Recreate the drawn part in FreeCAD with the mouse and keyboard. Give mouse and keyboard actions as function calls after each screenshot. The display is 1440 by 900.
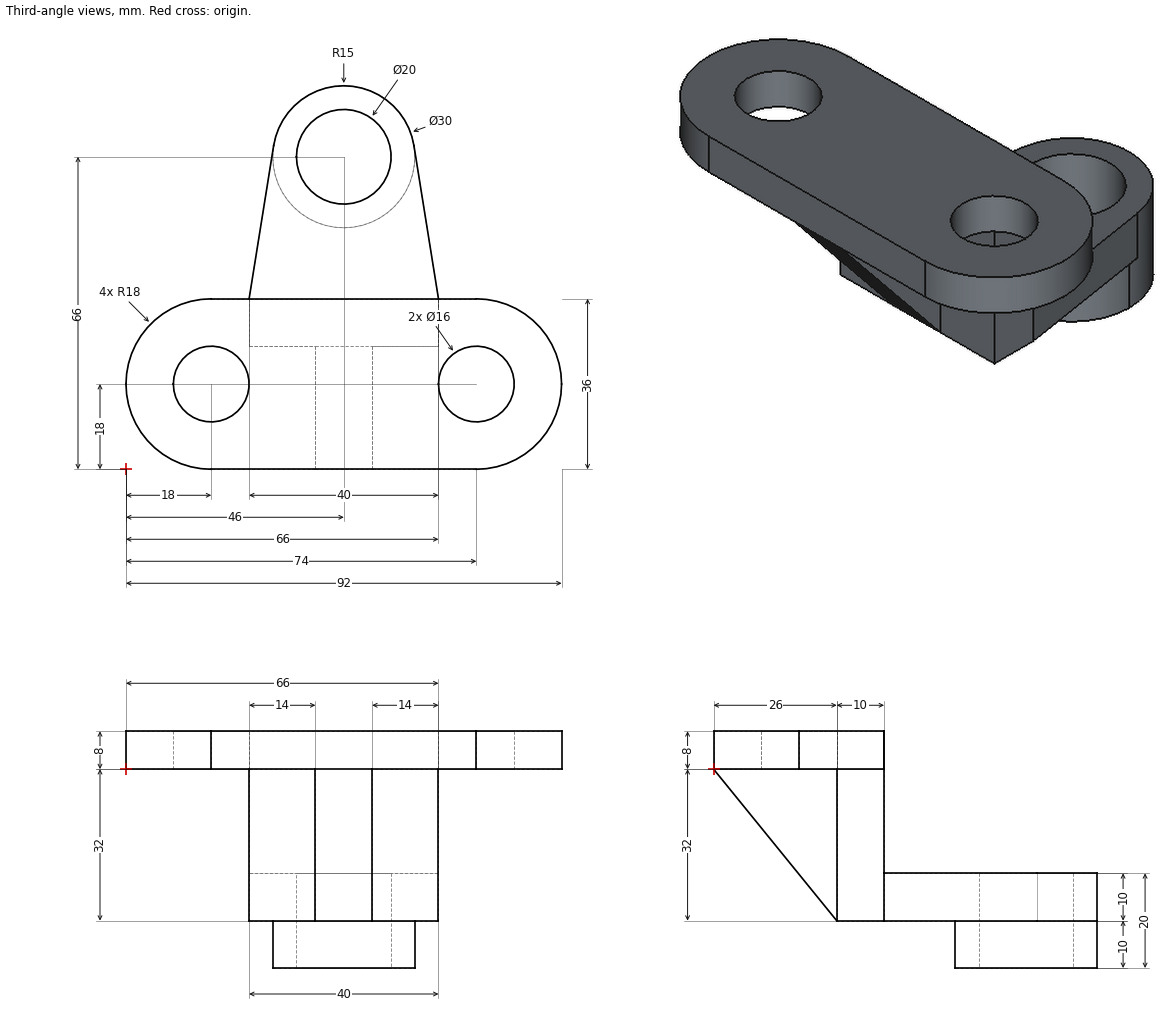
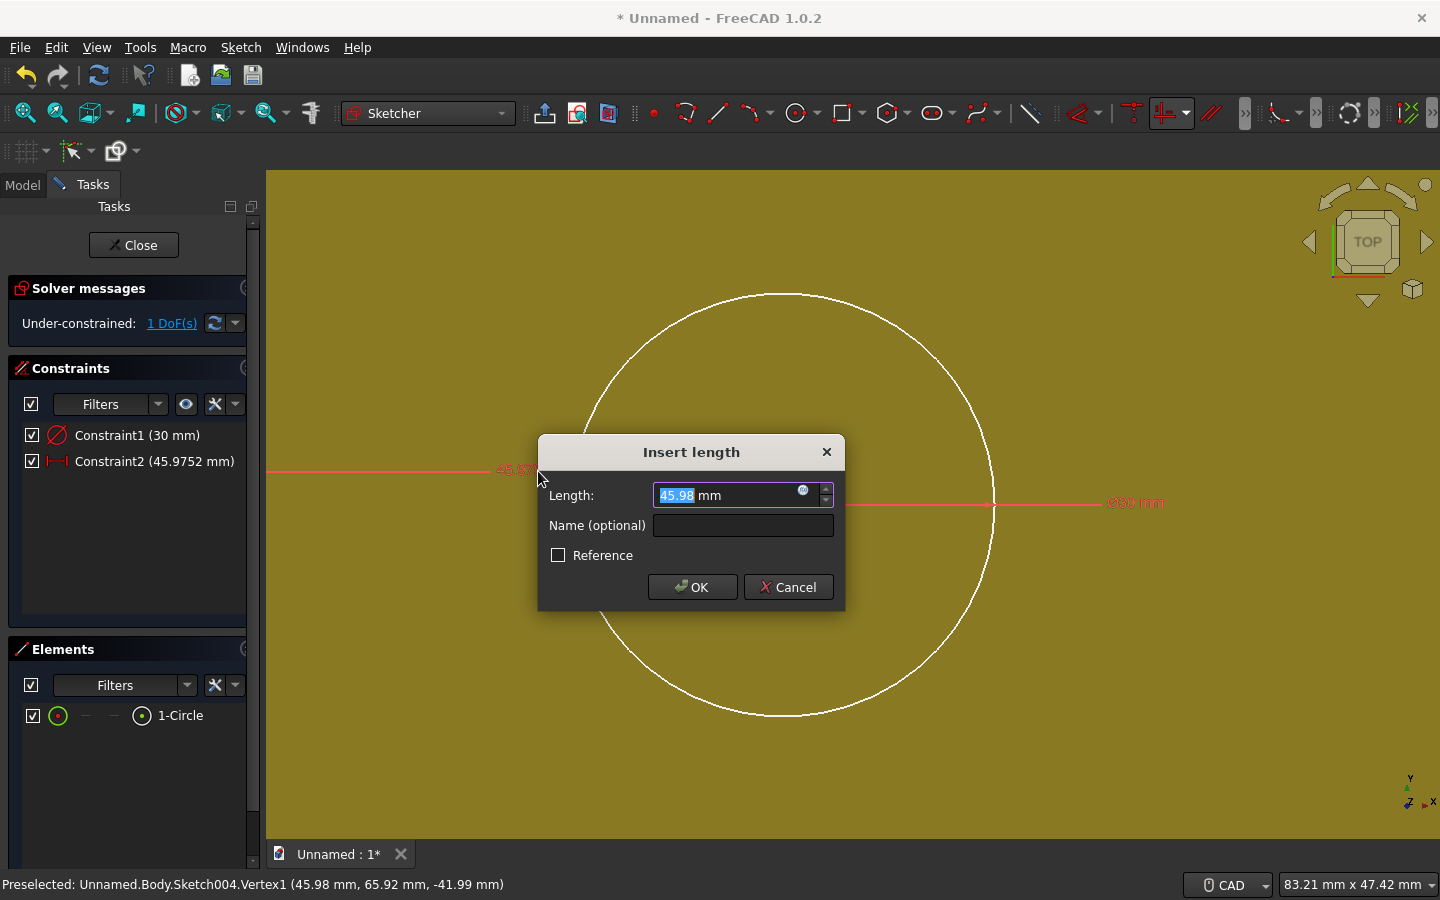
text(46)
key(Return)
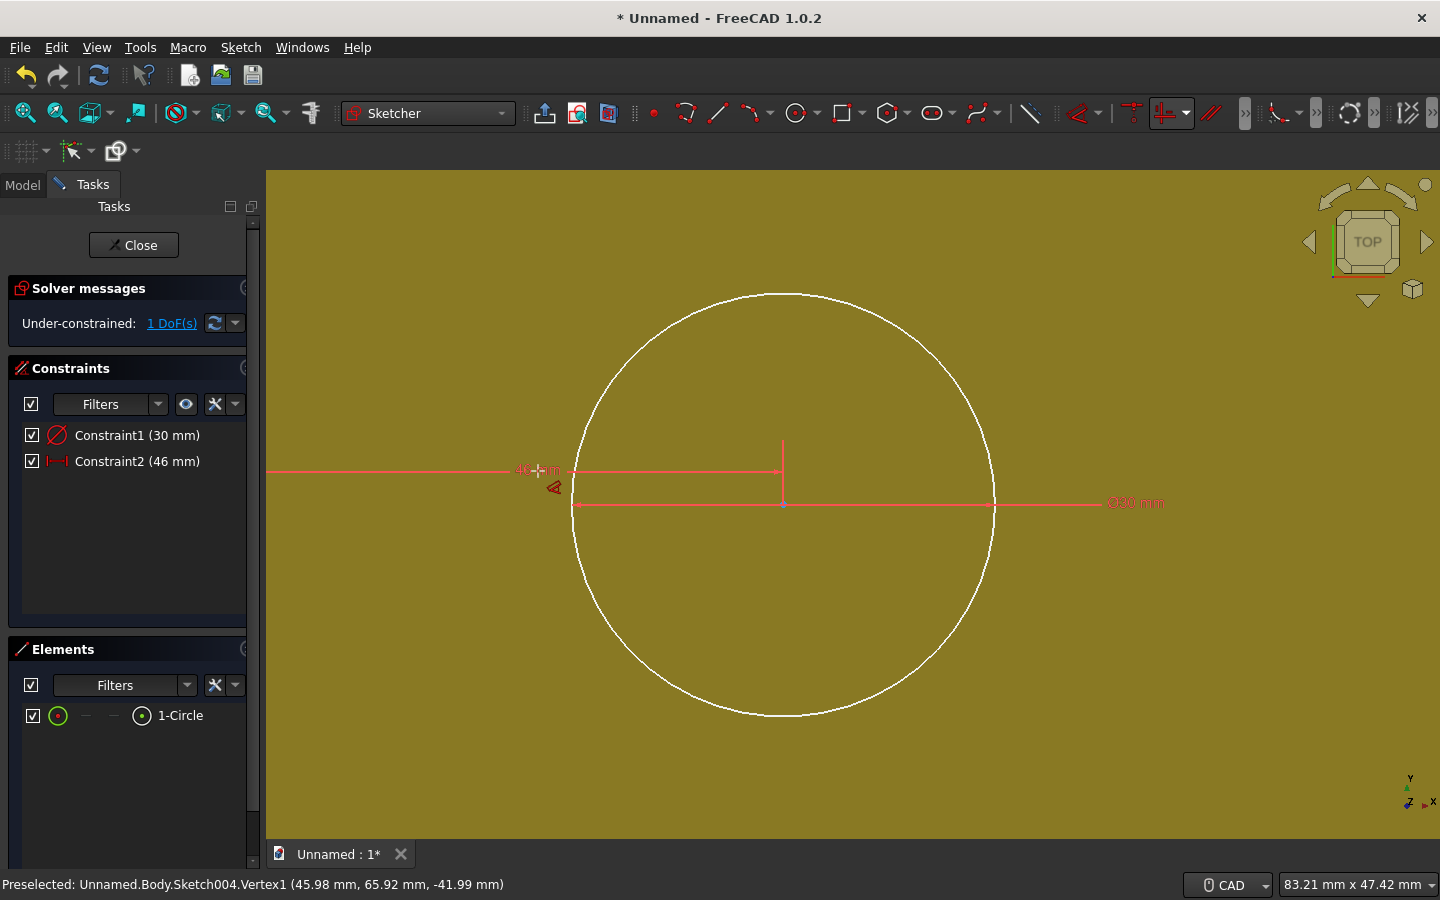
click(783, 505)
click(817, 658)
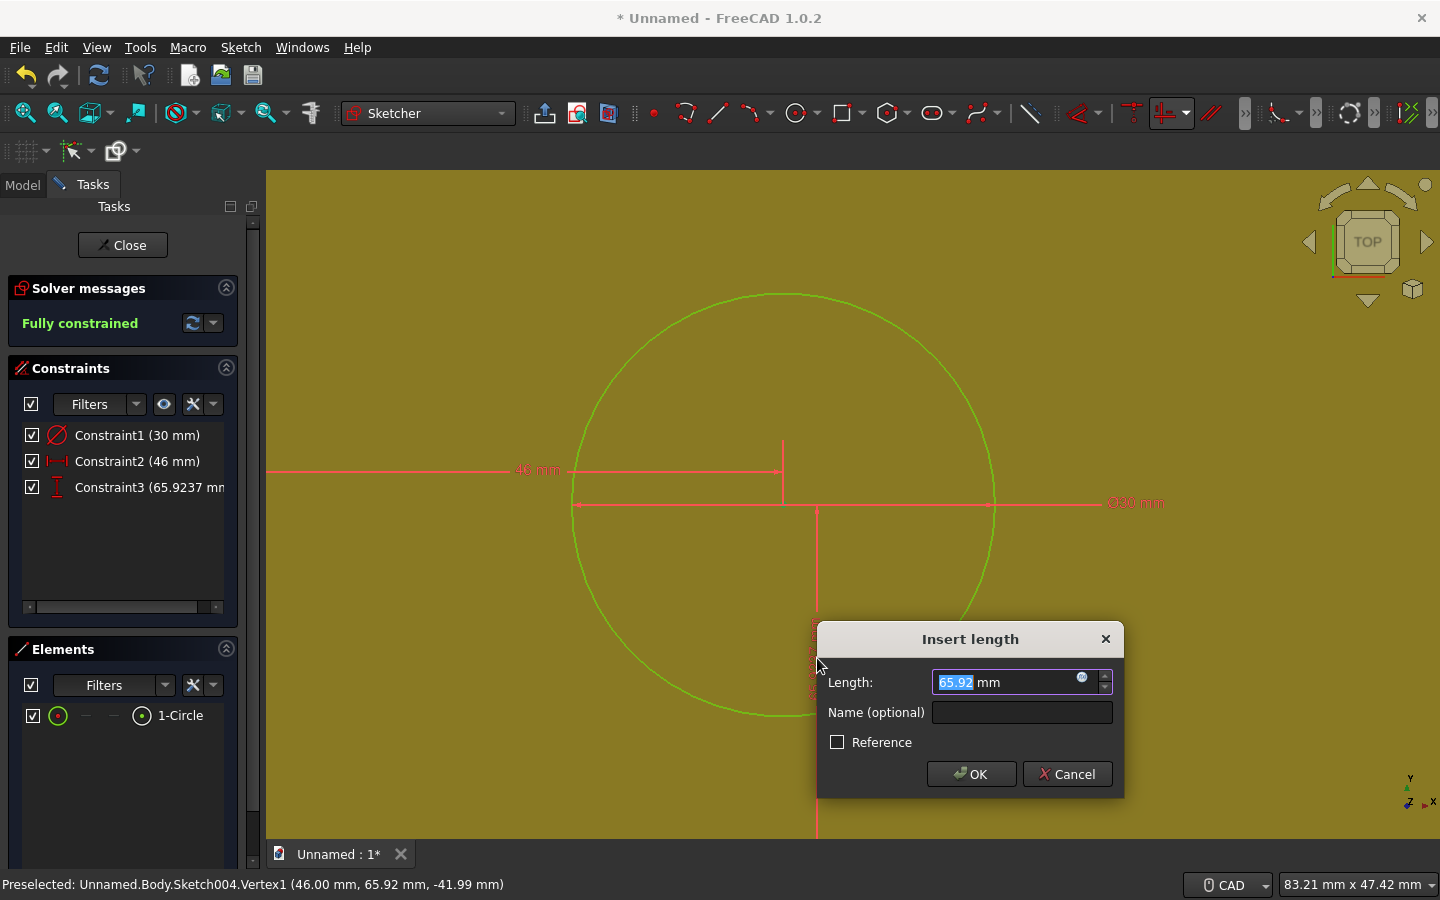
text(66)
key(Return)
key(Escape)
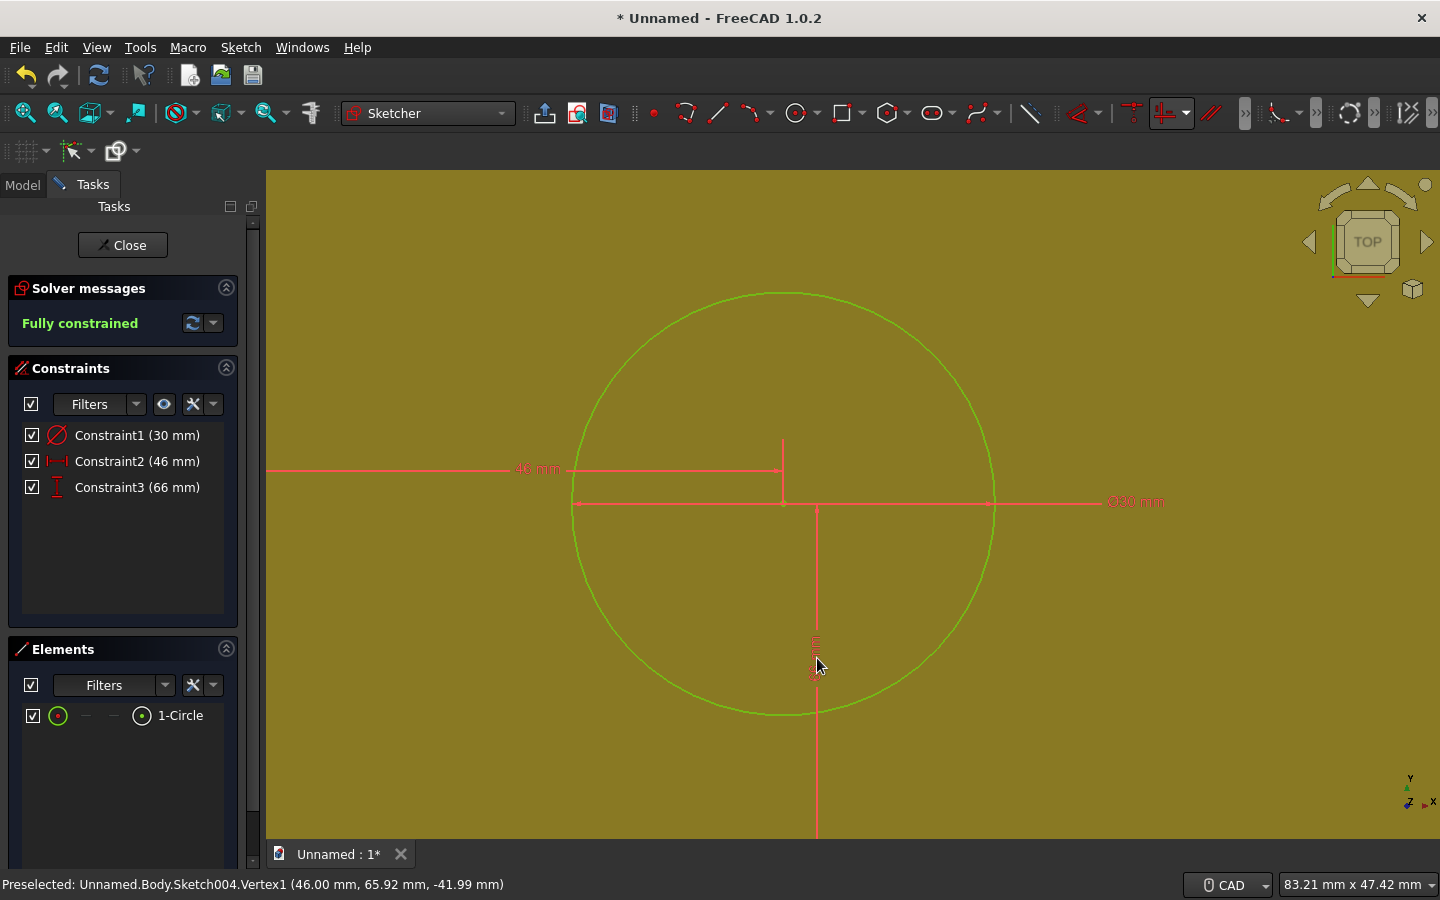
click(123, 245)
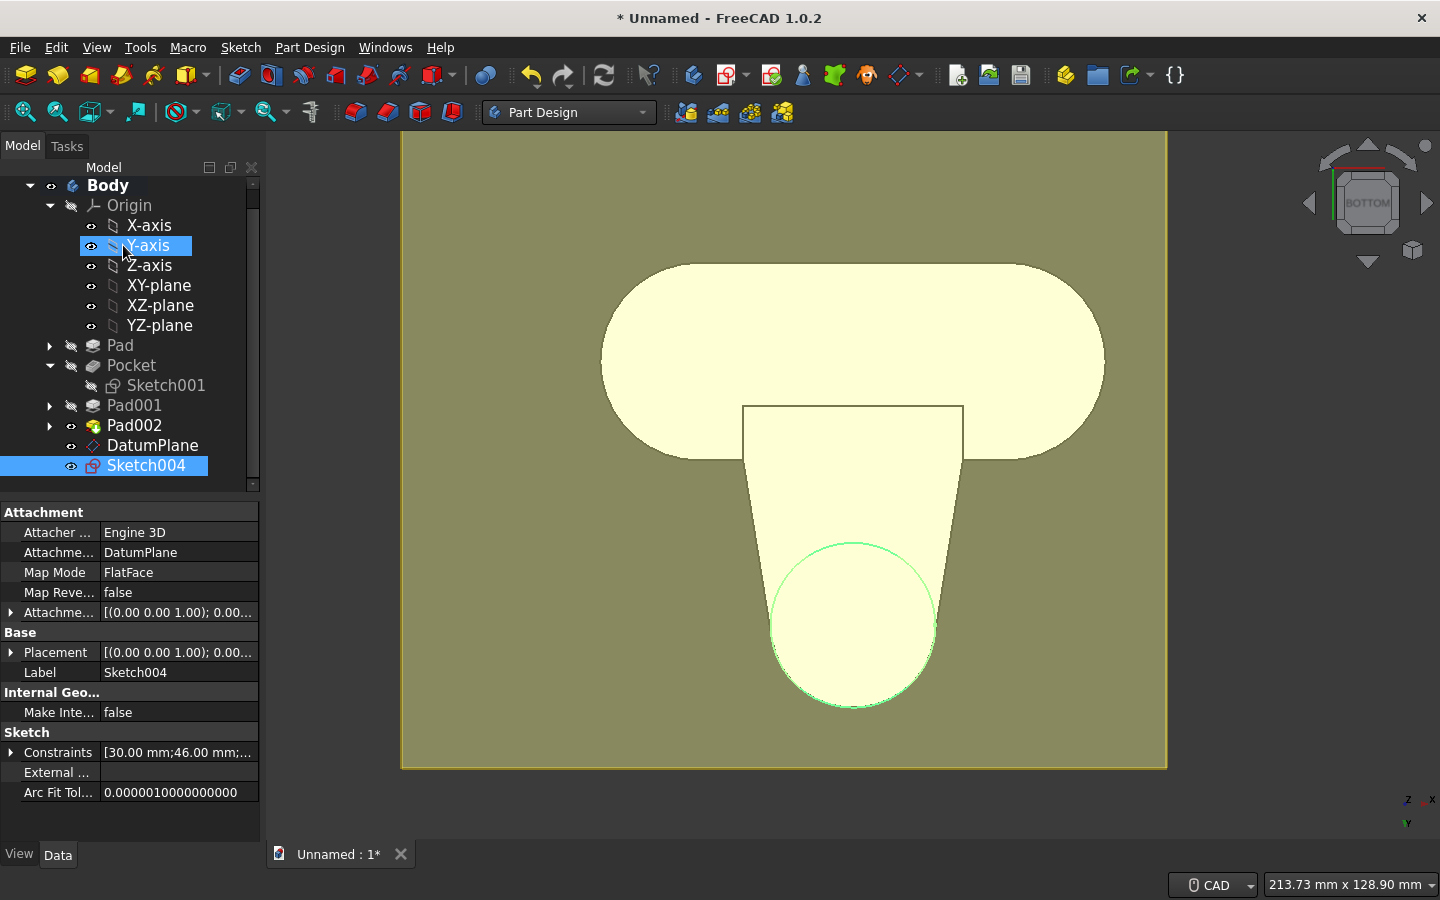
click(26, 76)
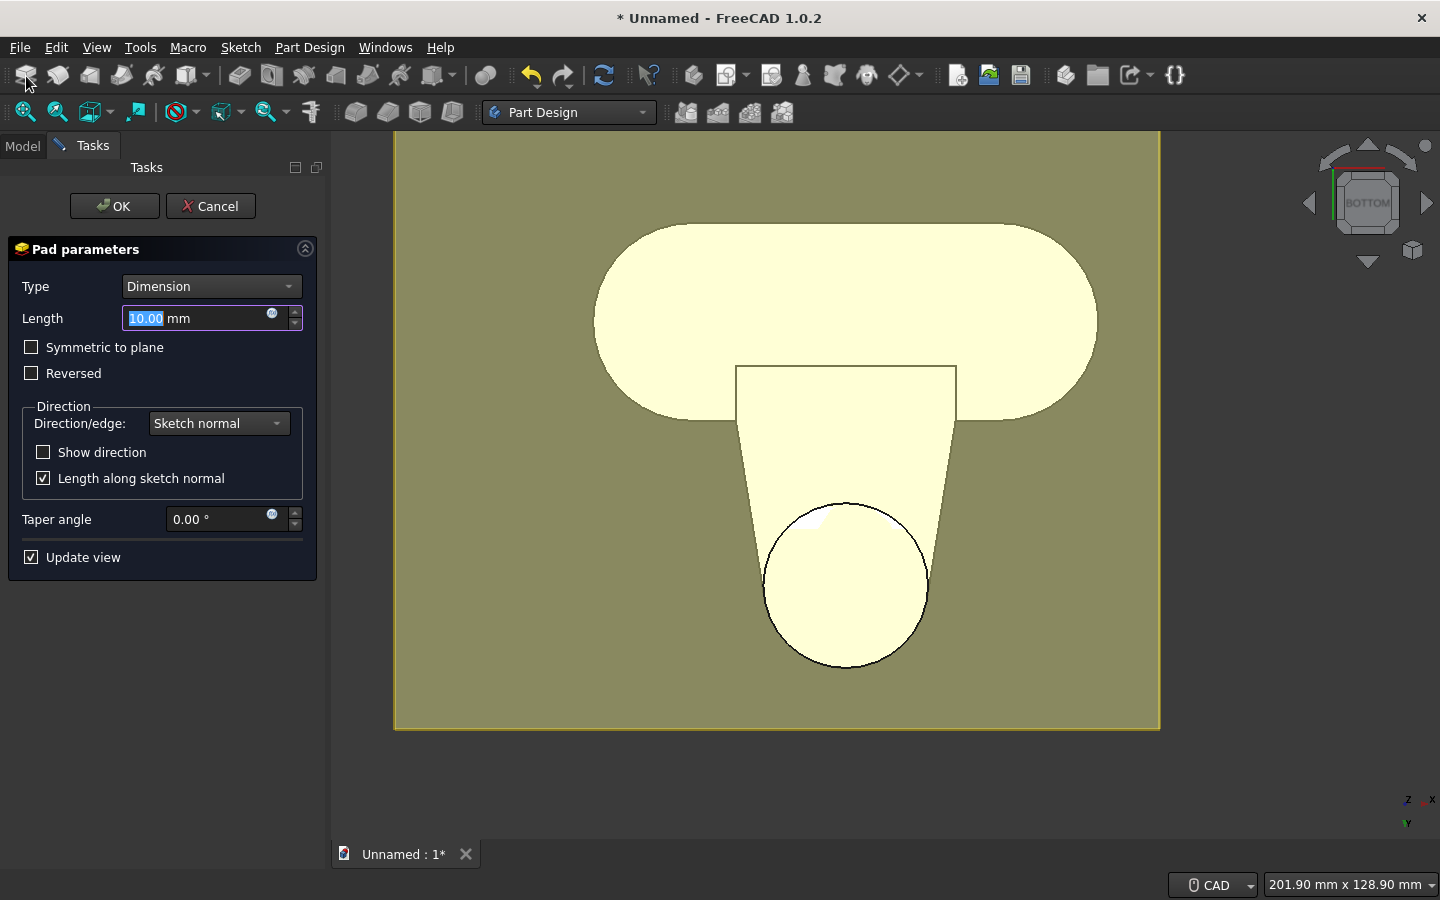
text(10)
key(Tab)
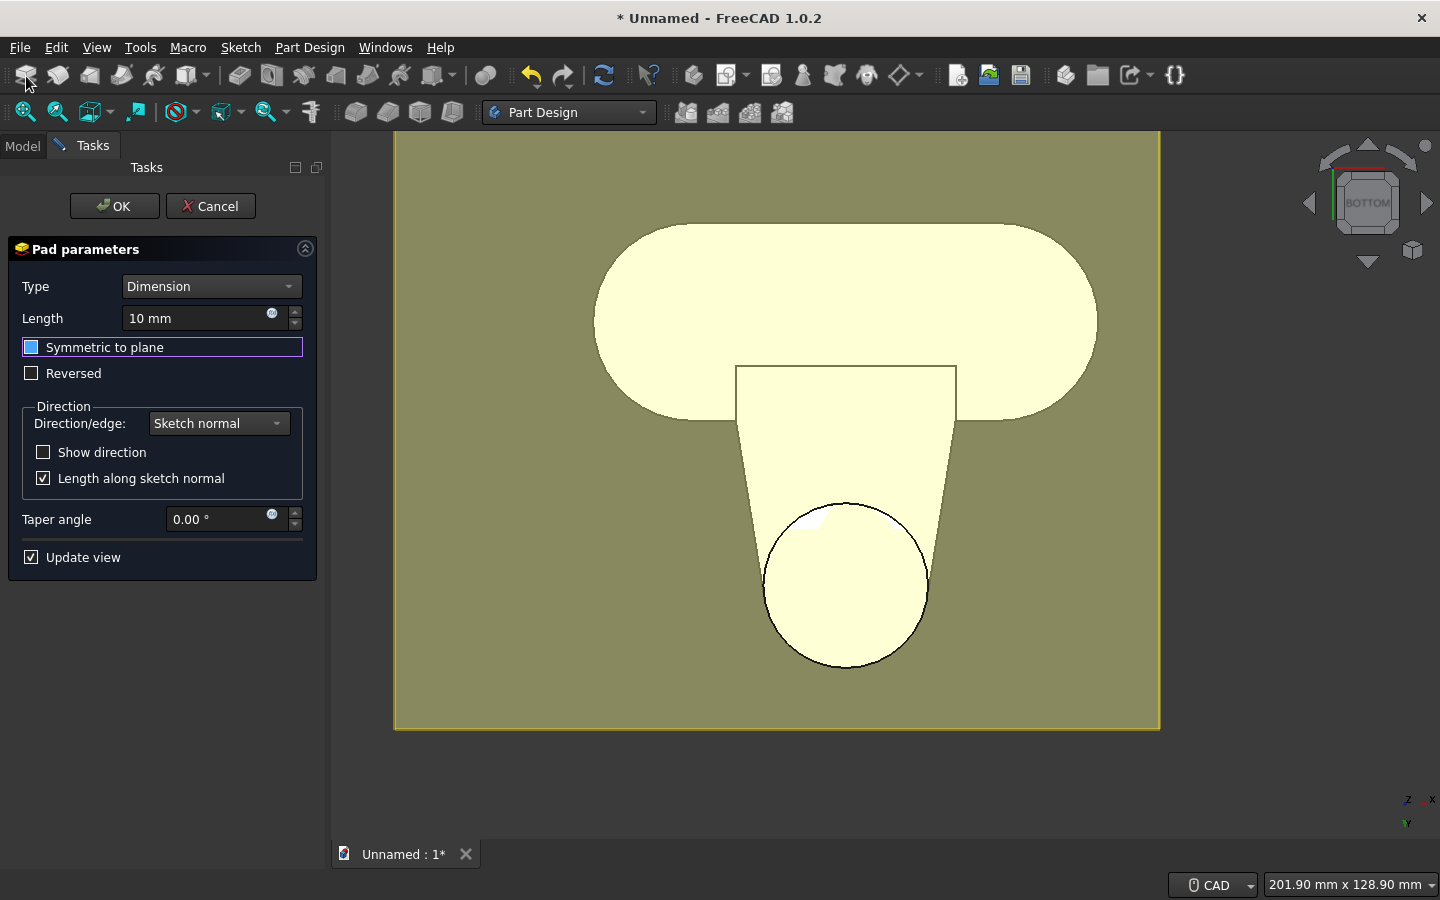
click(115, 206)